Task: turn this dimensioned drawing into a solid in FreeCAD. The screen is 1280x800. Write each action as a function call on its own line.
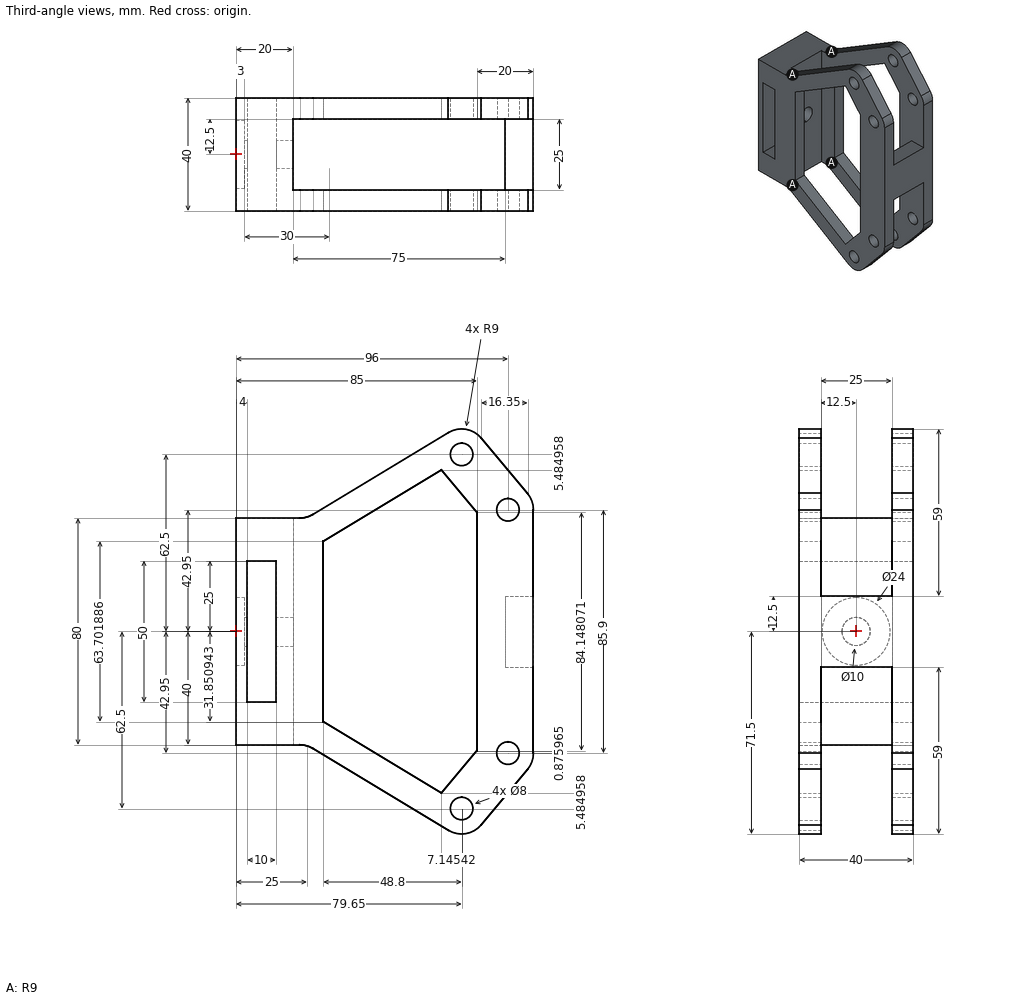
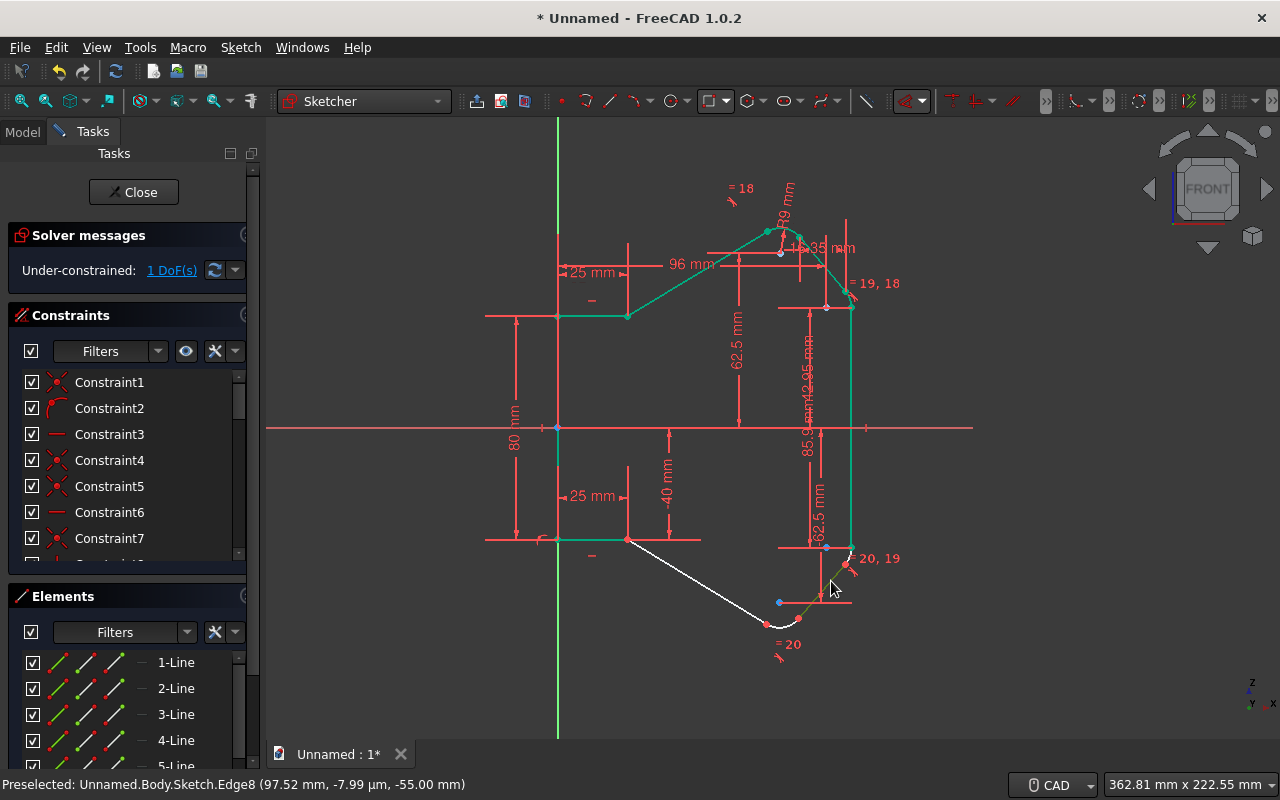
key(l)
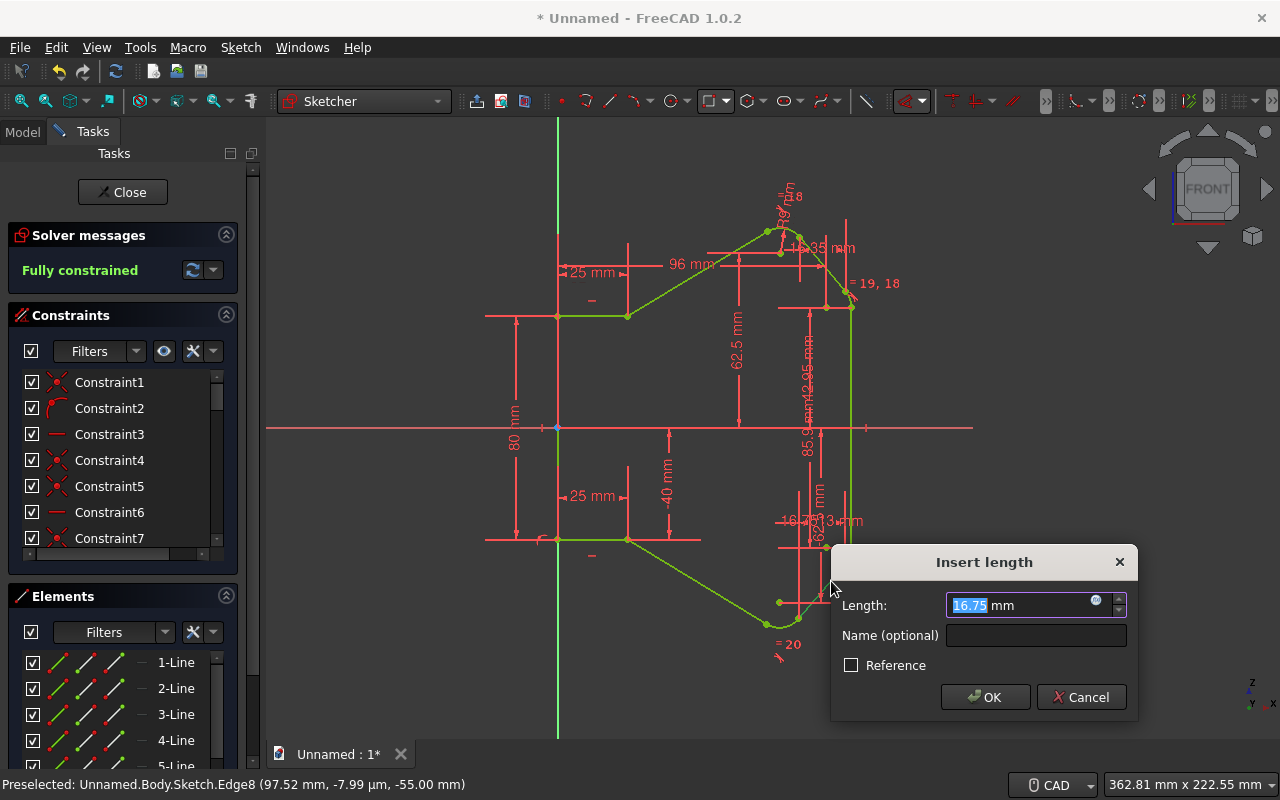
text(16.35)
key(Return)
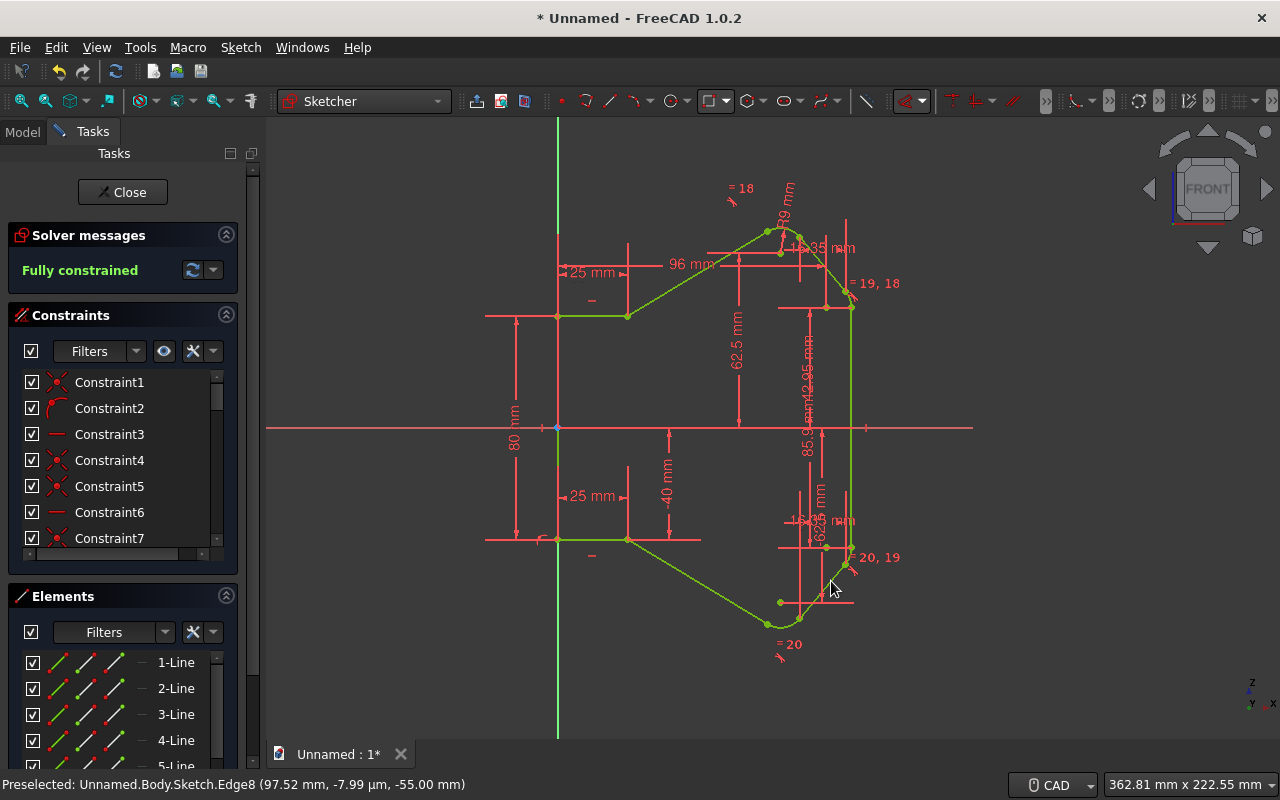
click(123, 192)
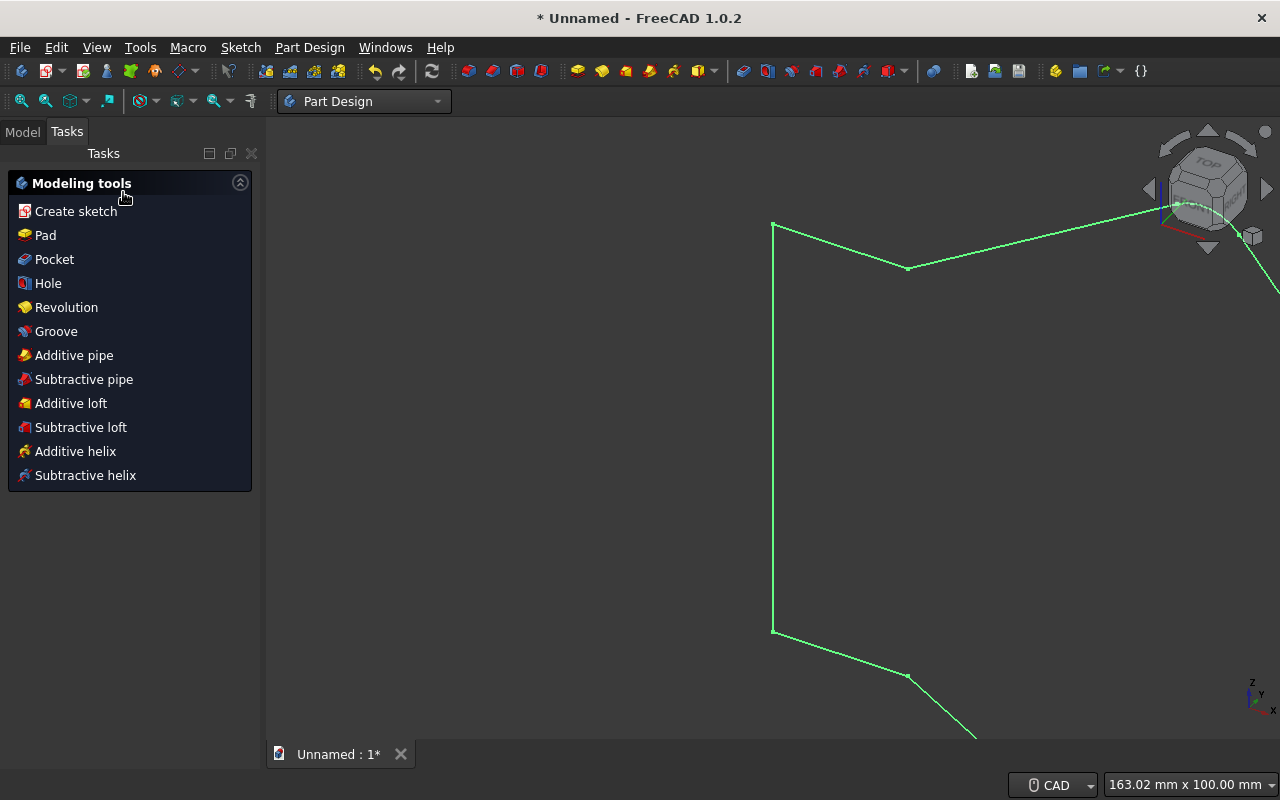
click(578, 72)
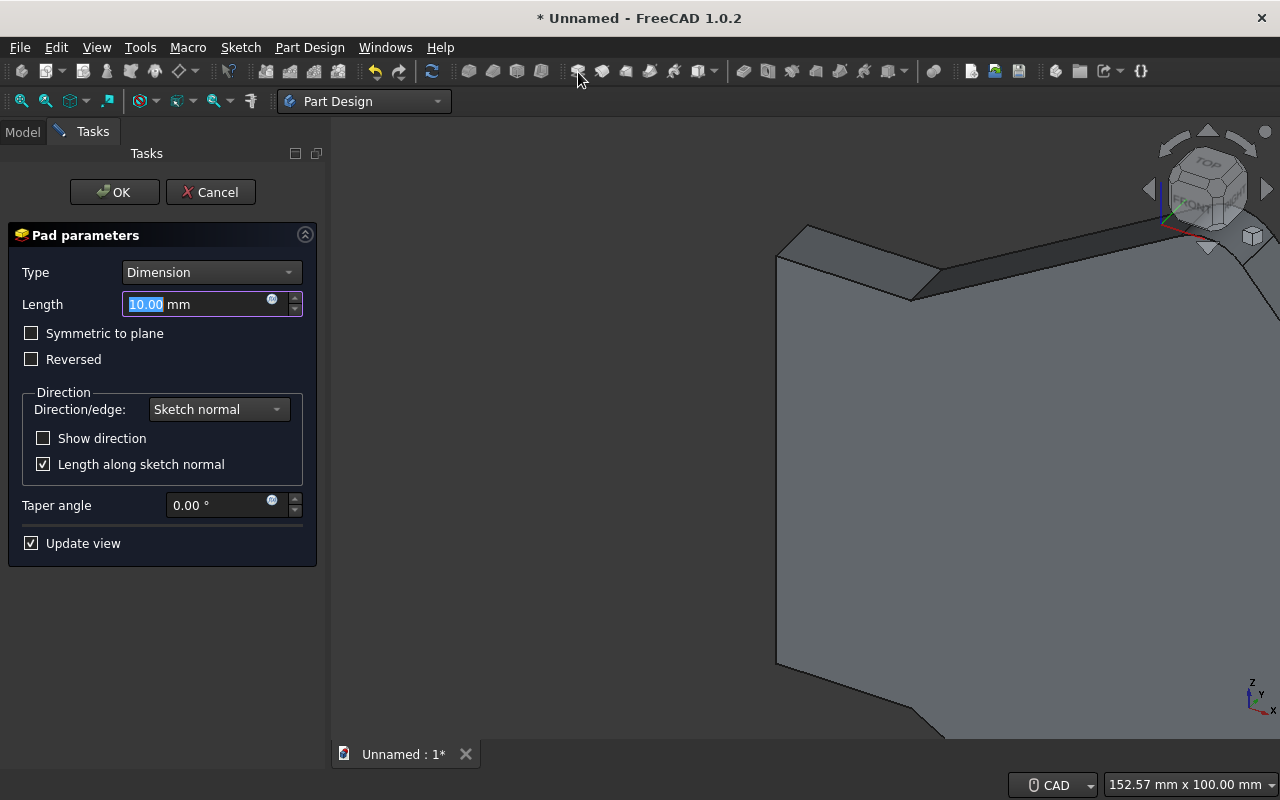
text(40)
key(Tab)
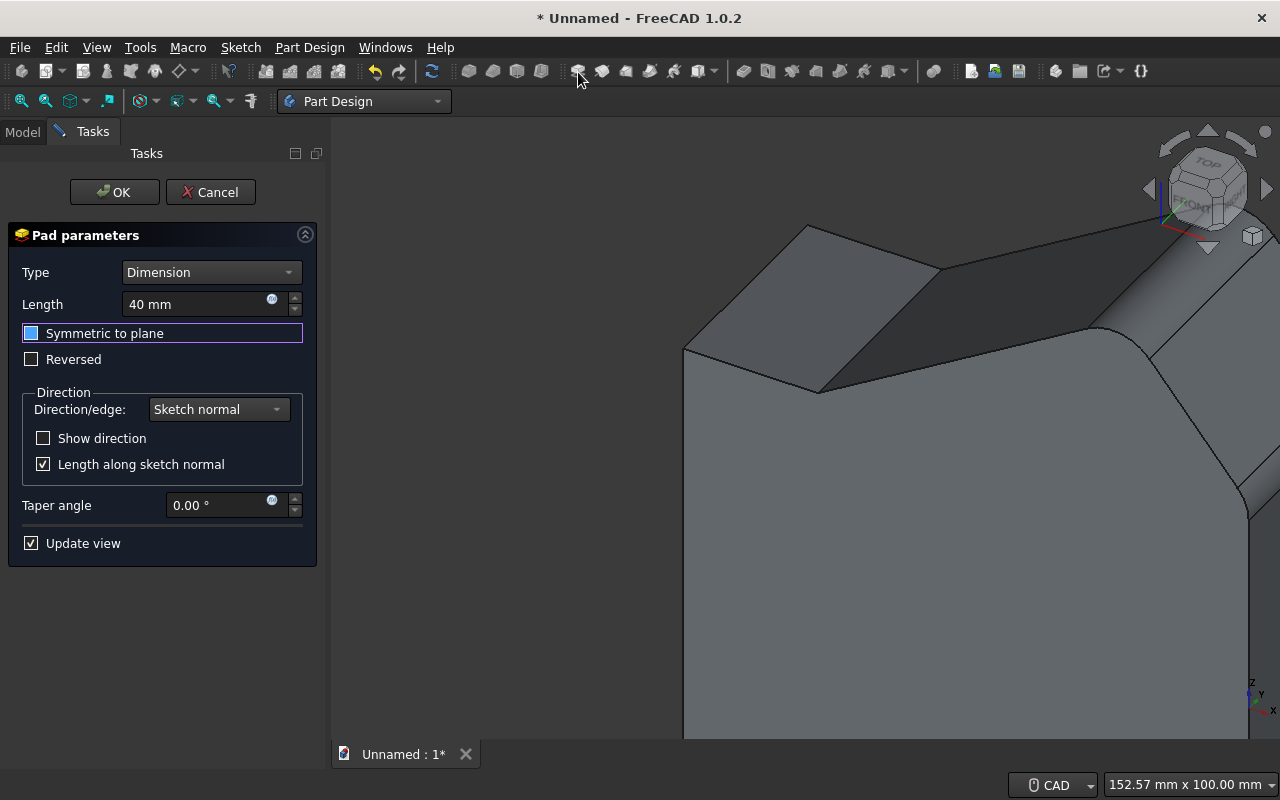
click(30, 333)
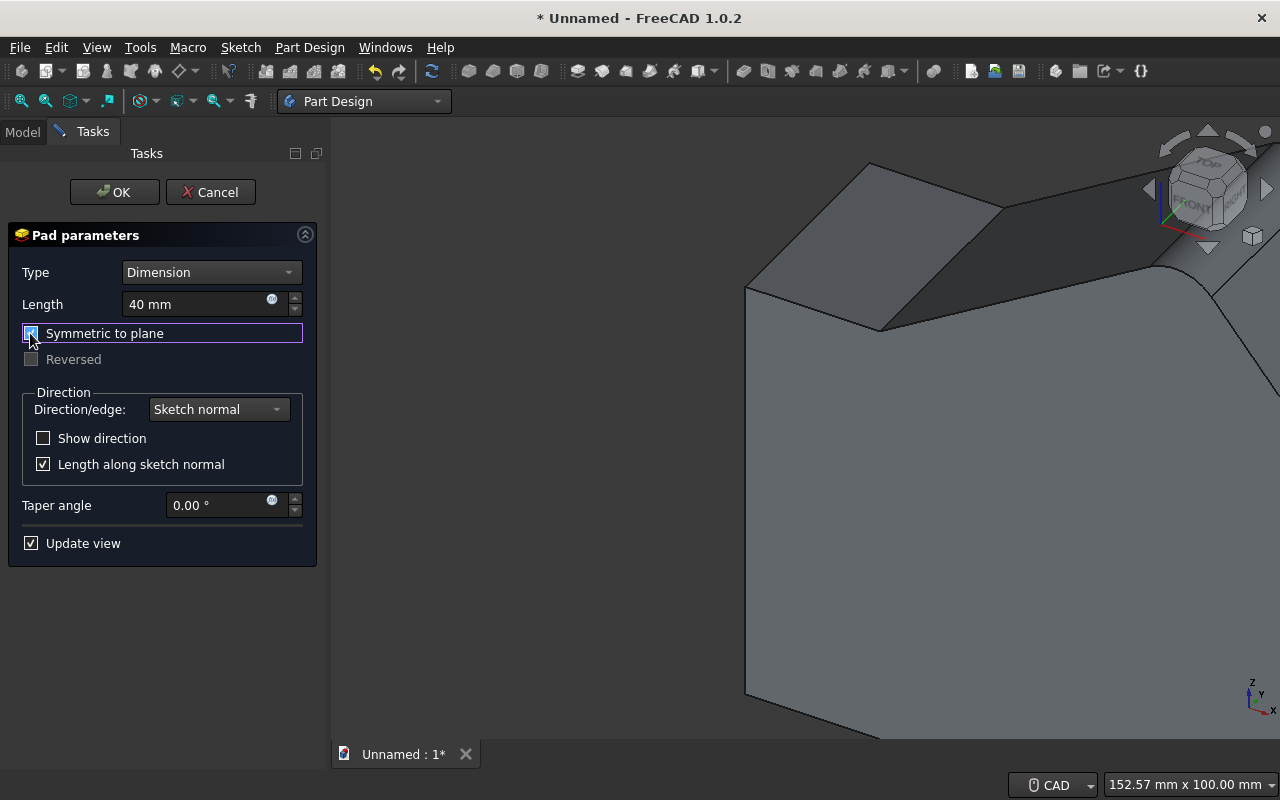
click(115, 192)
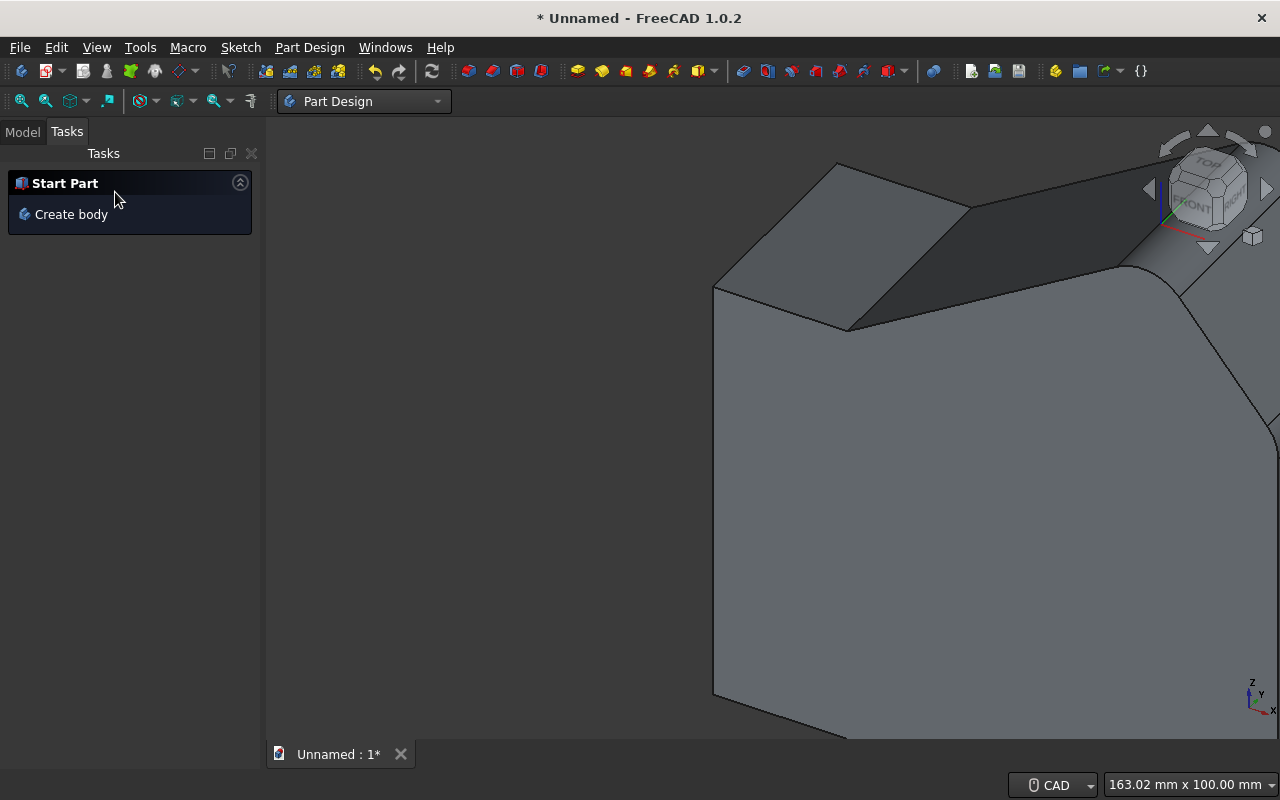
key(v)
key(f)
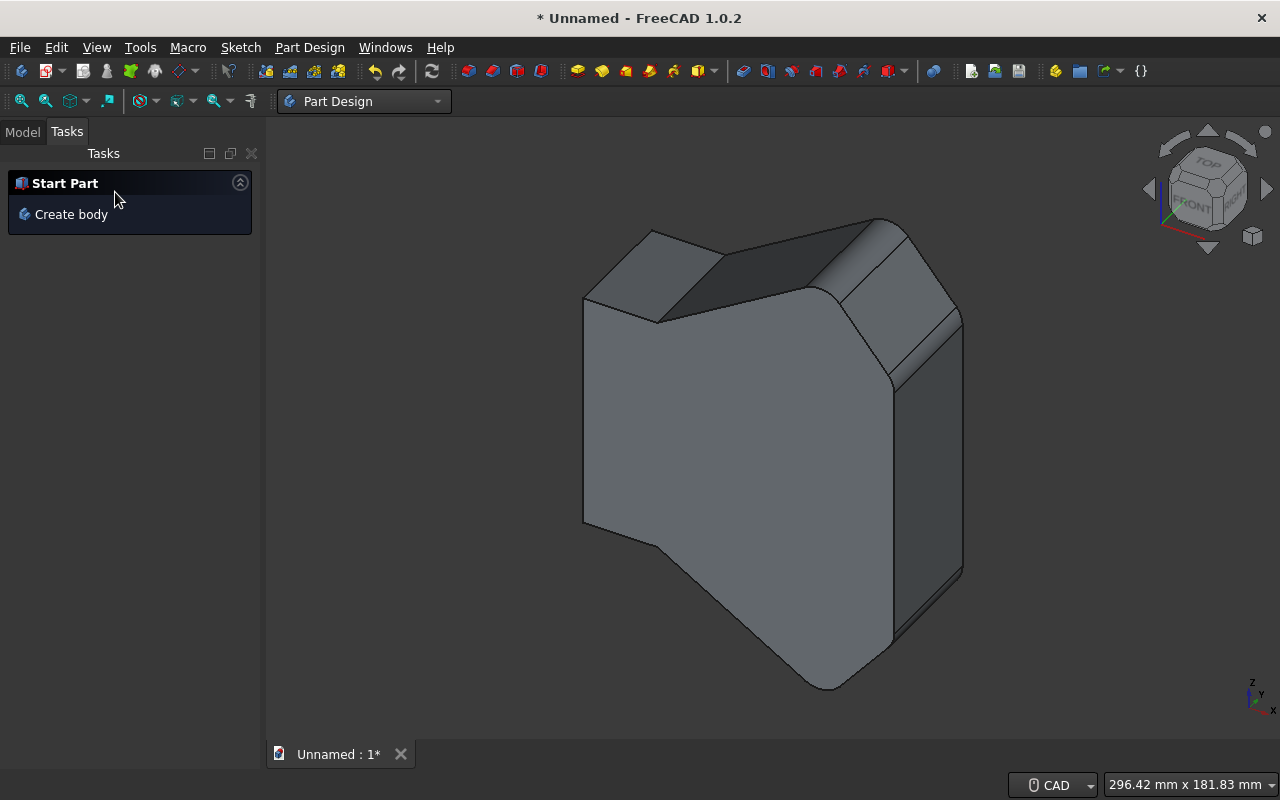
click(46, 72)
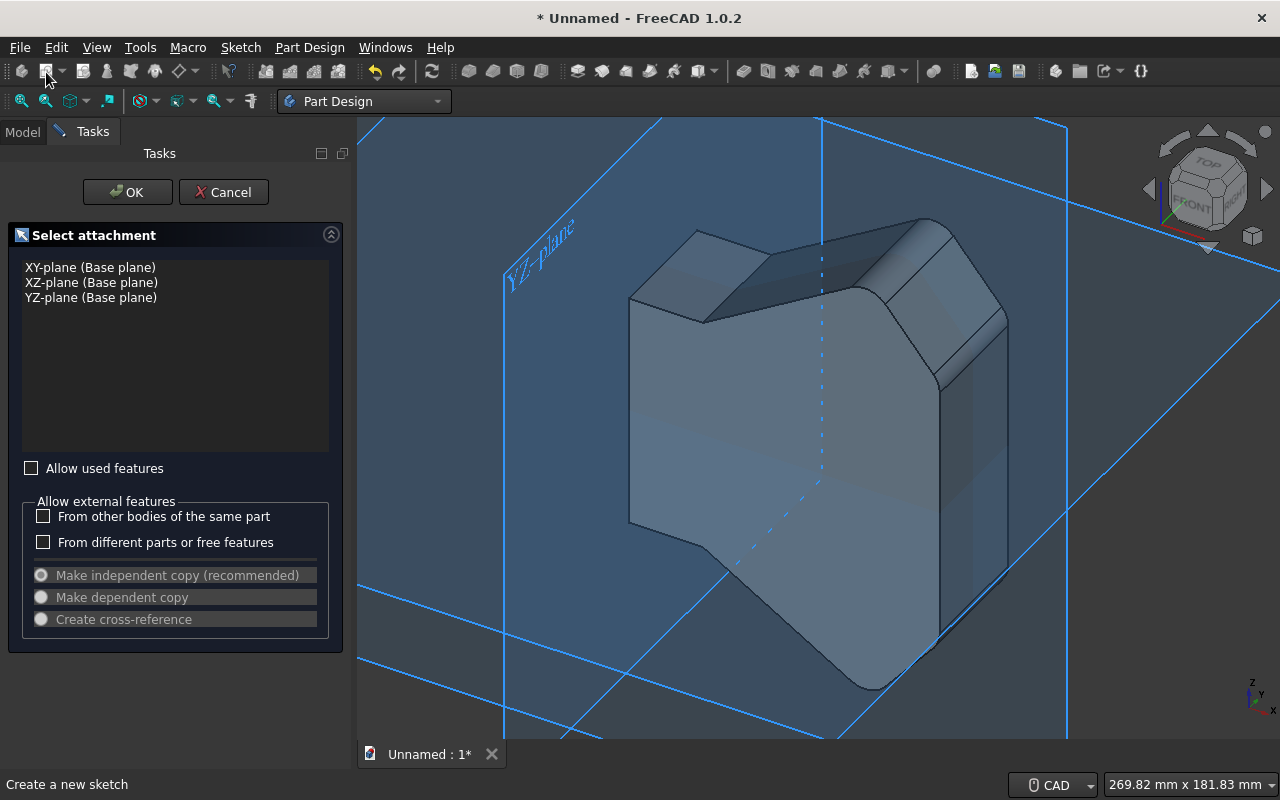
click(82, 282)